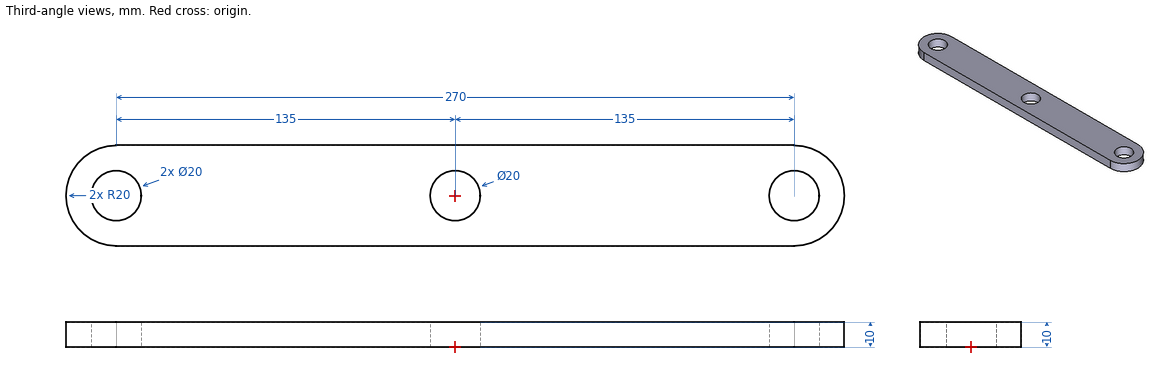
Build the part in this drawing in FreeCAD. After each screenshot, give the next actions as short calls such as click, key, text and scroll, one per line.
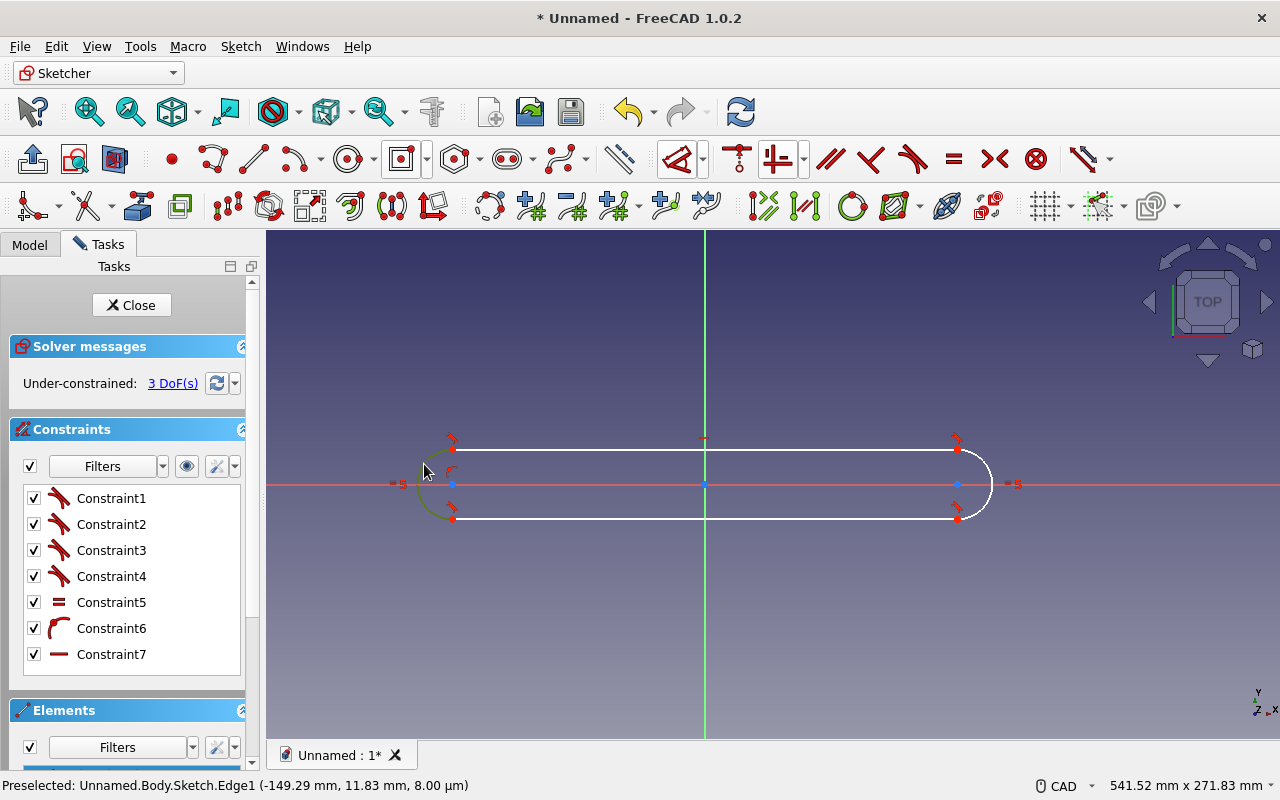
click(702, 160)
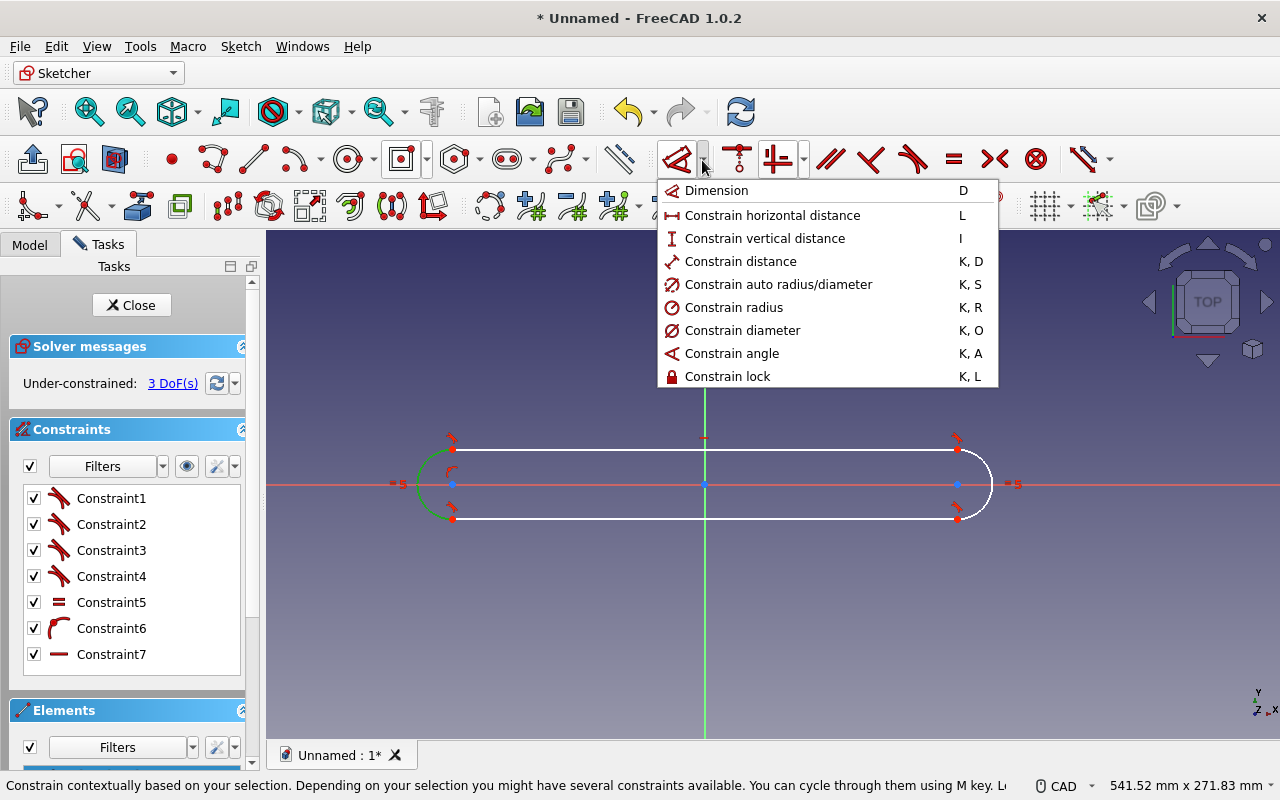
click(828, 308)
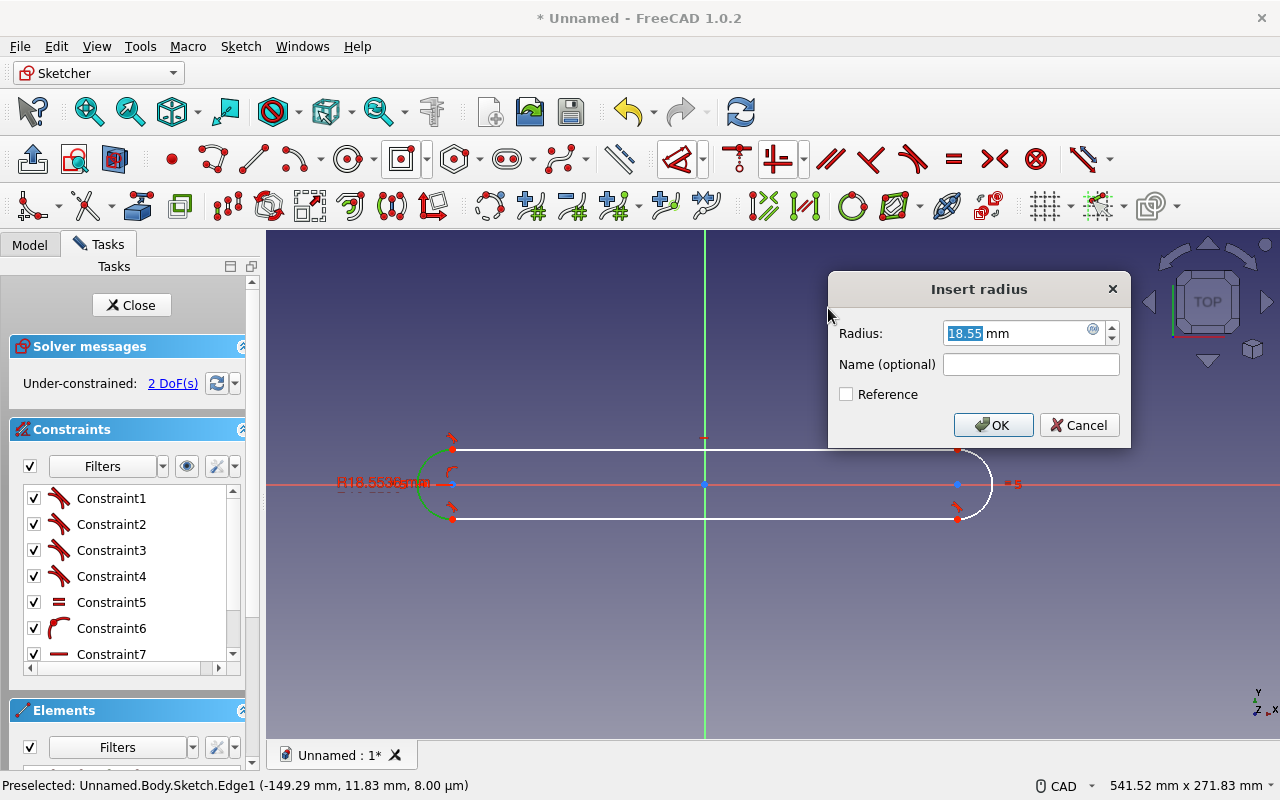
text(20)
key(Return)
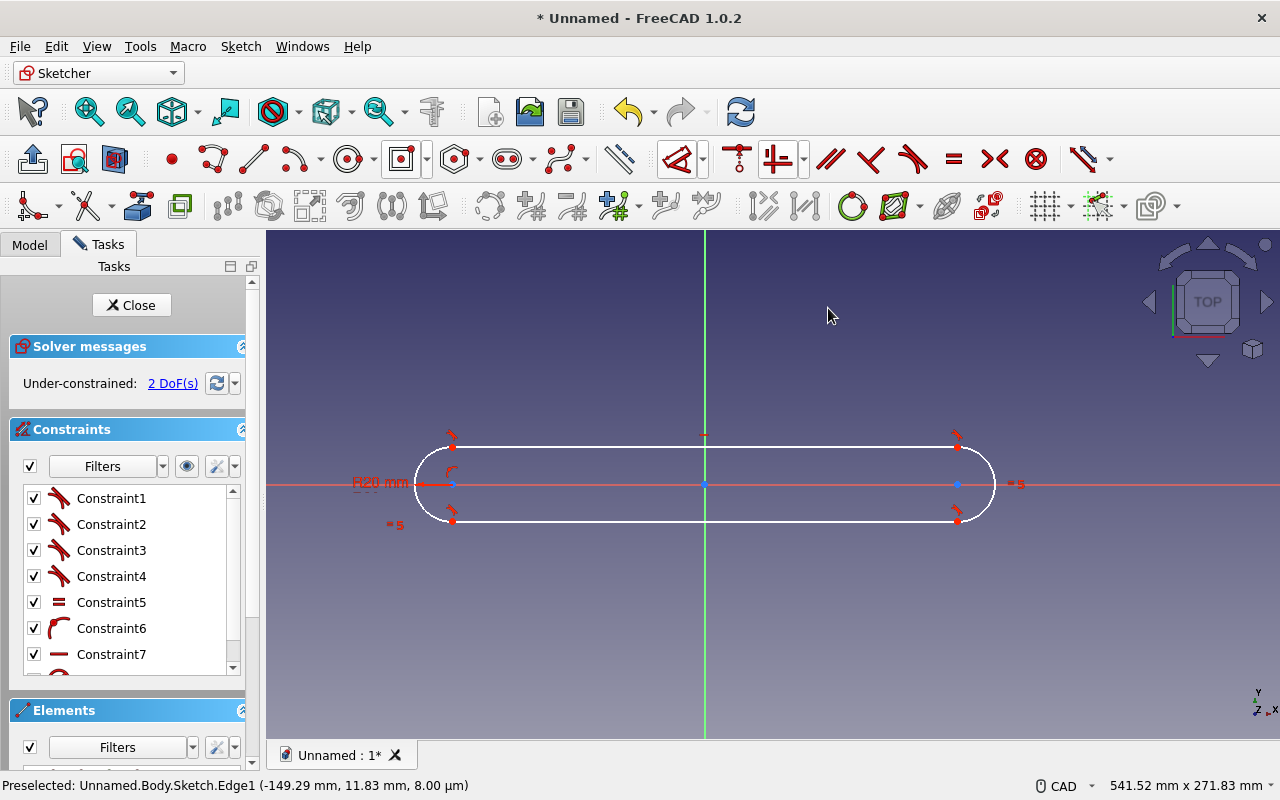
click(604, 447)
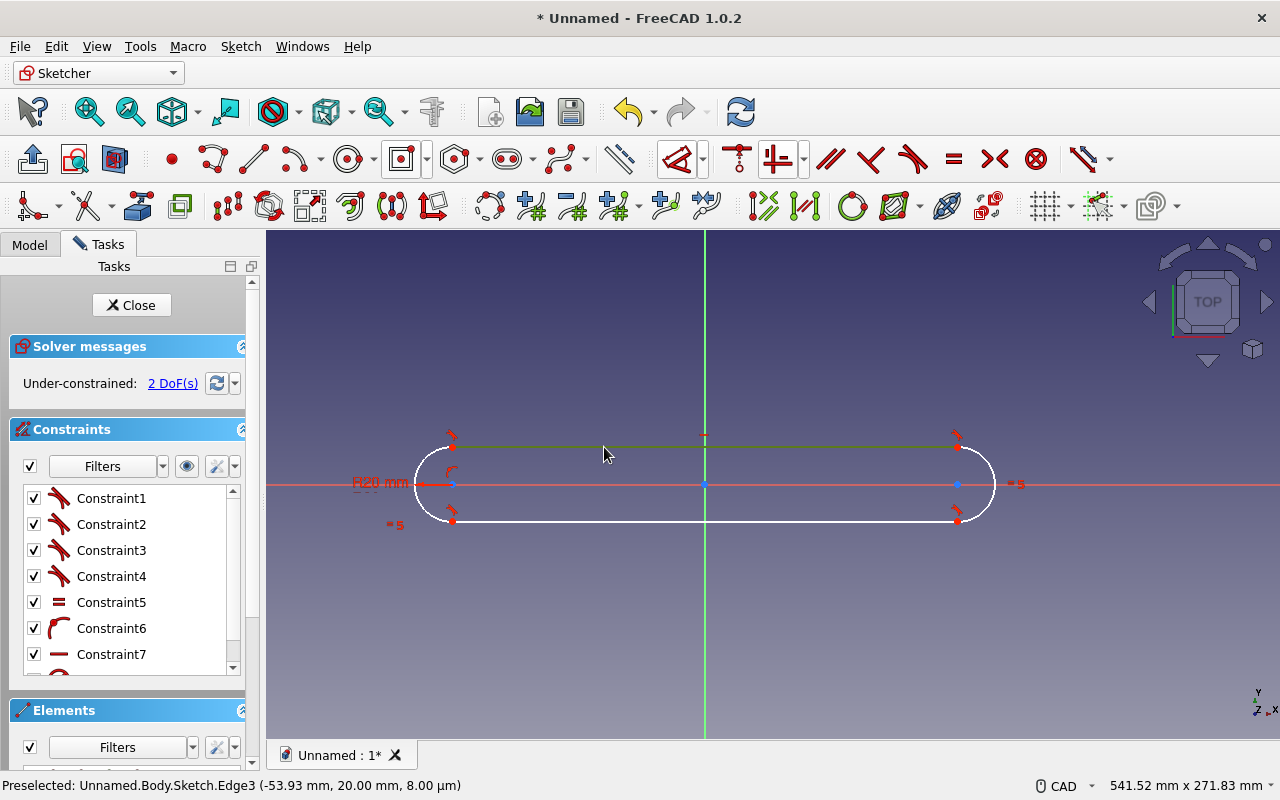
key(l)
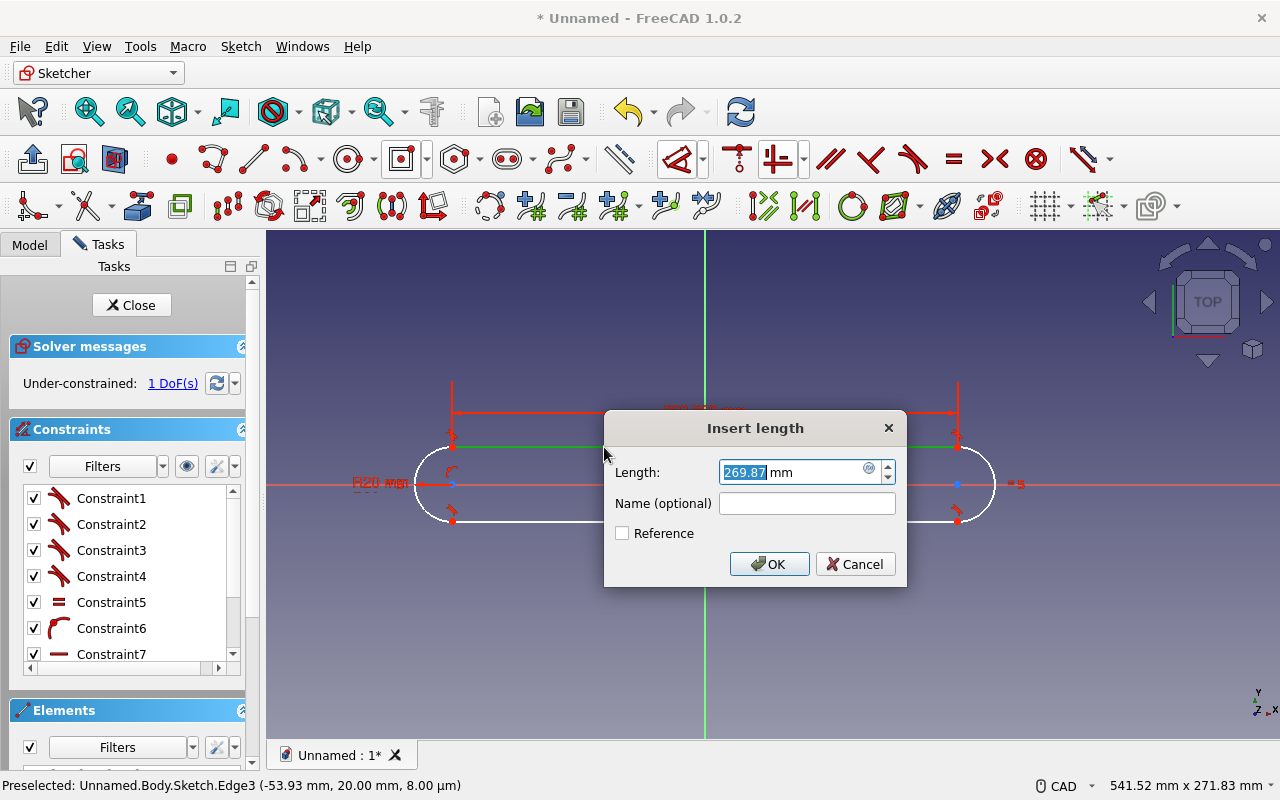
text(270)
key(Return)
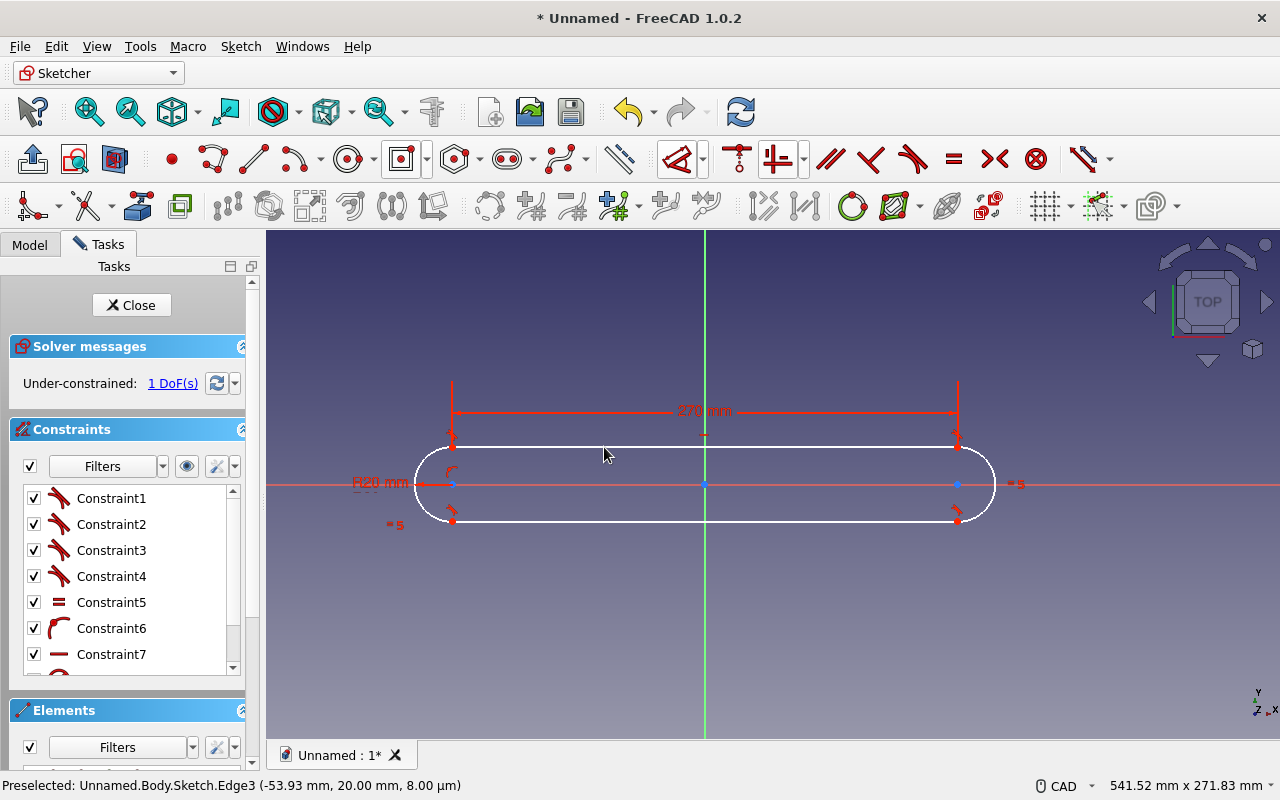
click(452, 447)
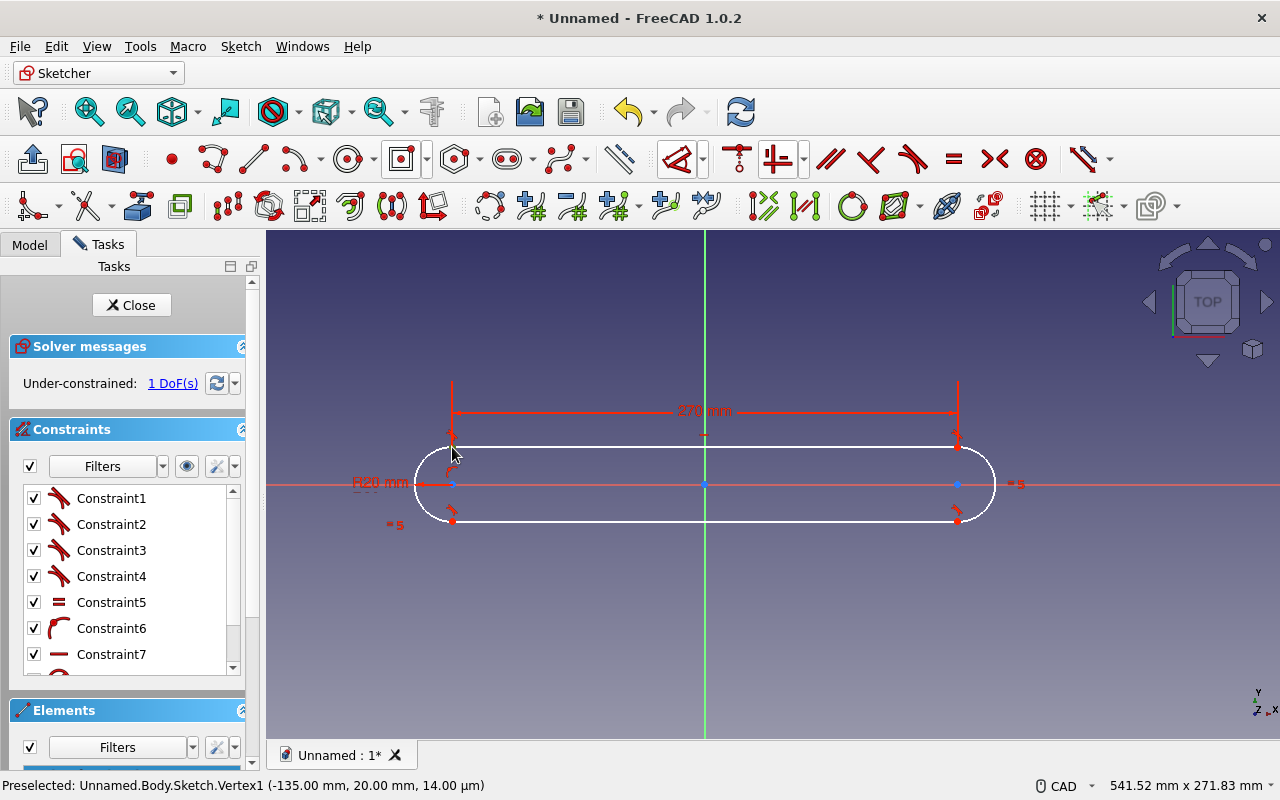
key(l)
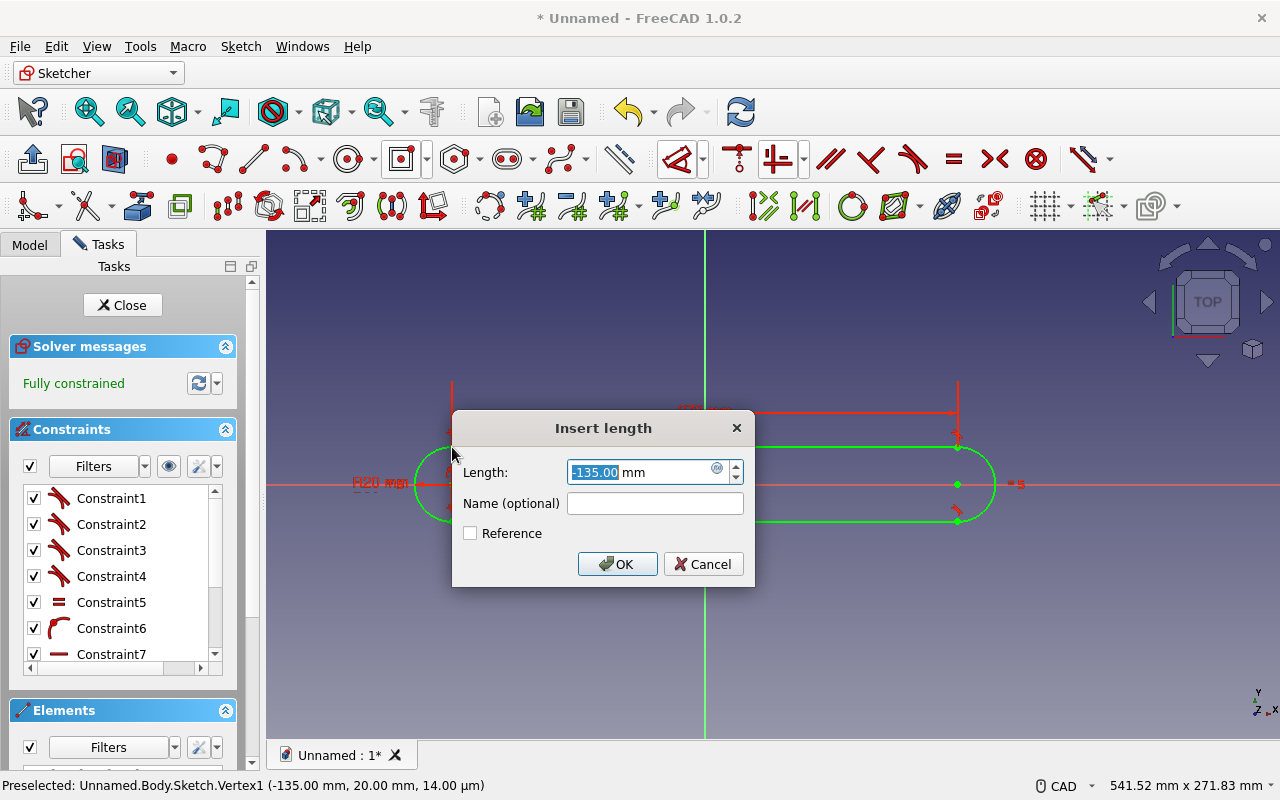
text(-135)
key(Return)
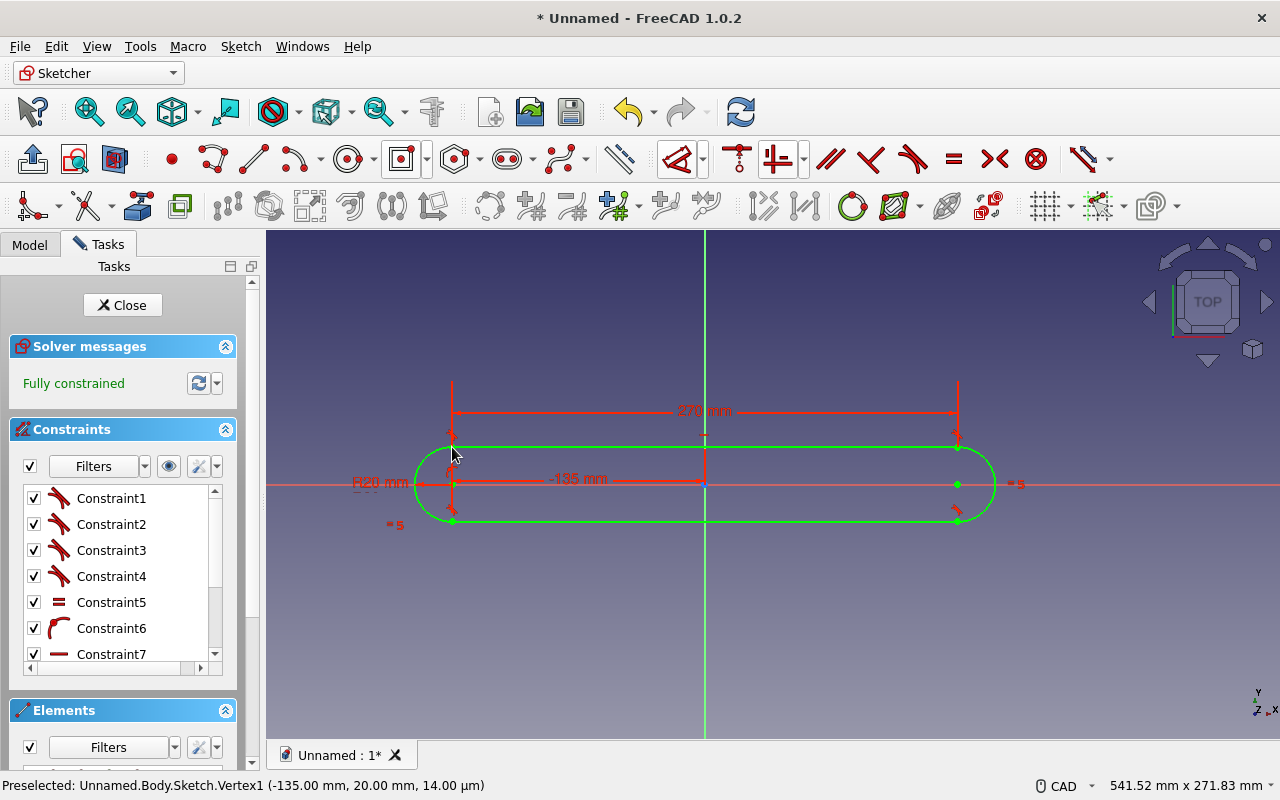
click(123, 305)